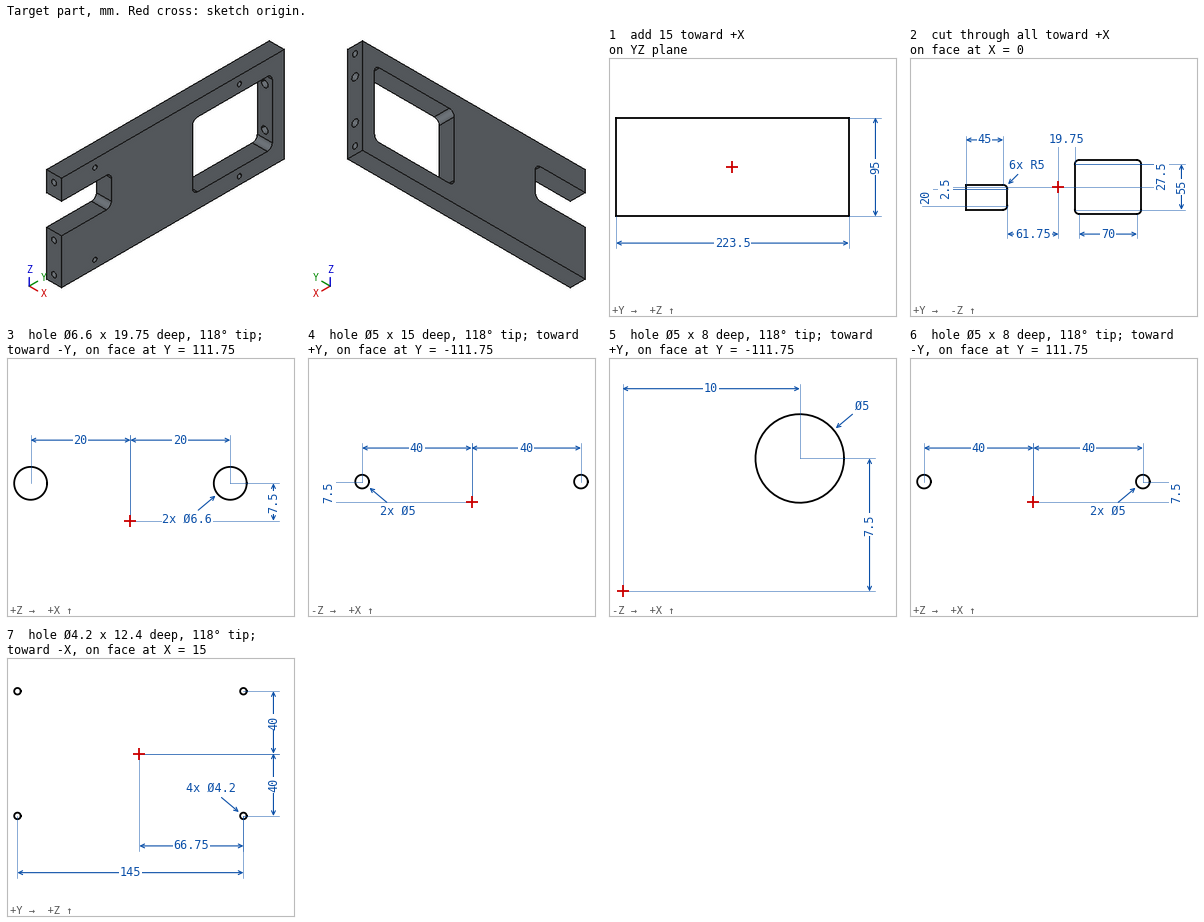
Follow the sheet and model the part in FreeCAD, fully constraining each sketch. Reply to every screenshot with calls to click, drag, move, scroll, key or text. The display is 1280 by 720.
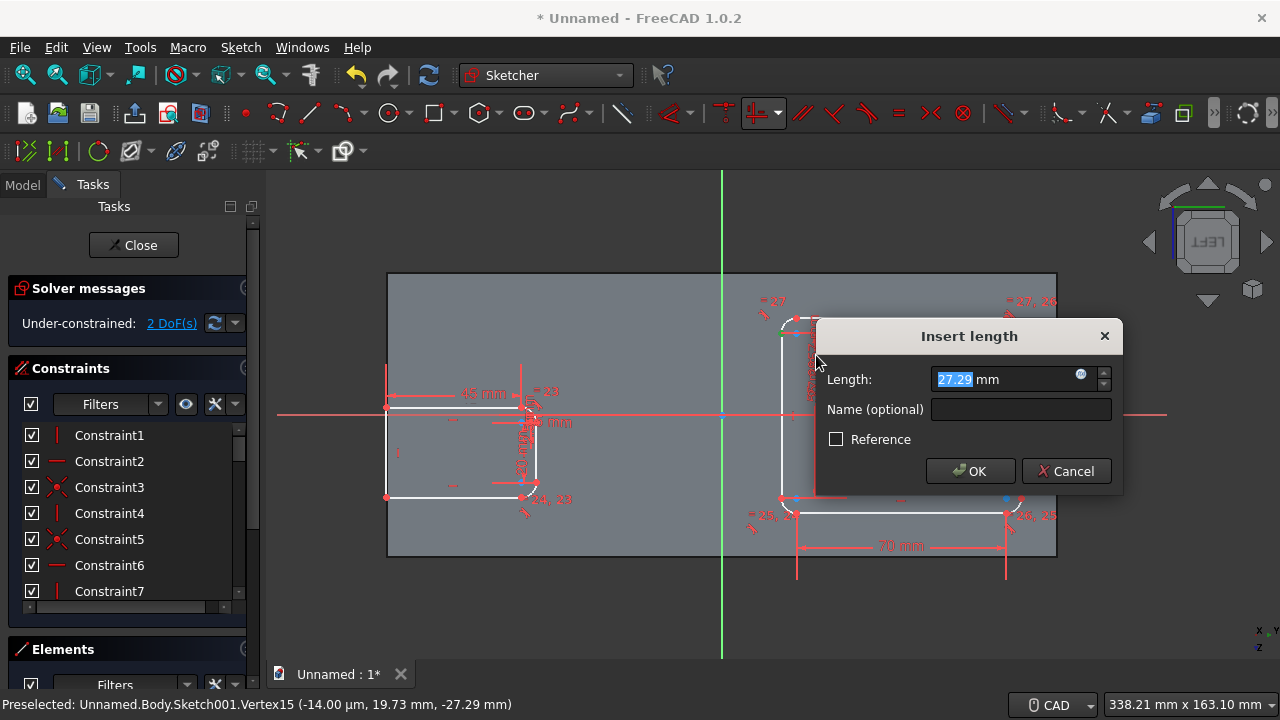
text(27.5)
key(Return)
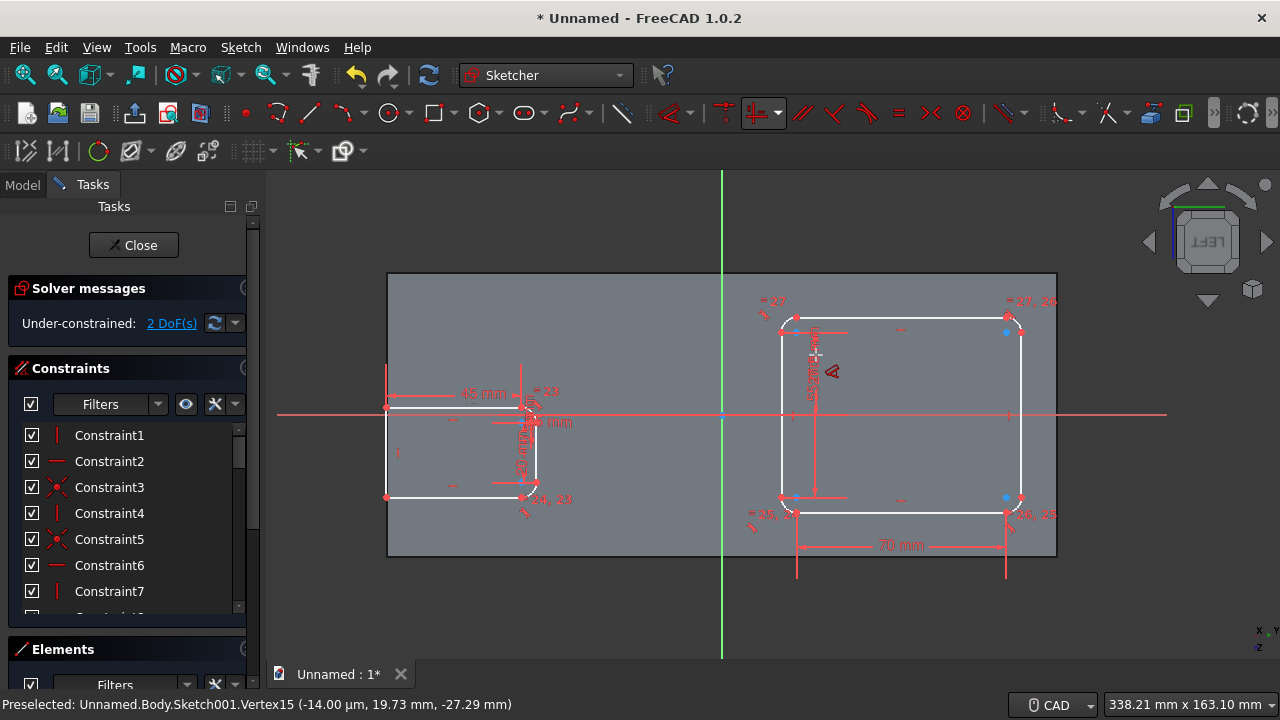
click(536, 483)
click(629, 517)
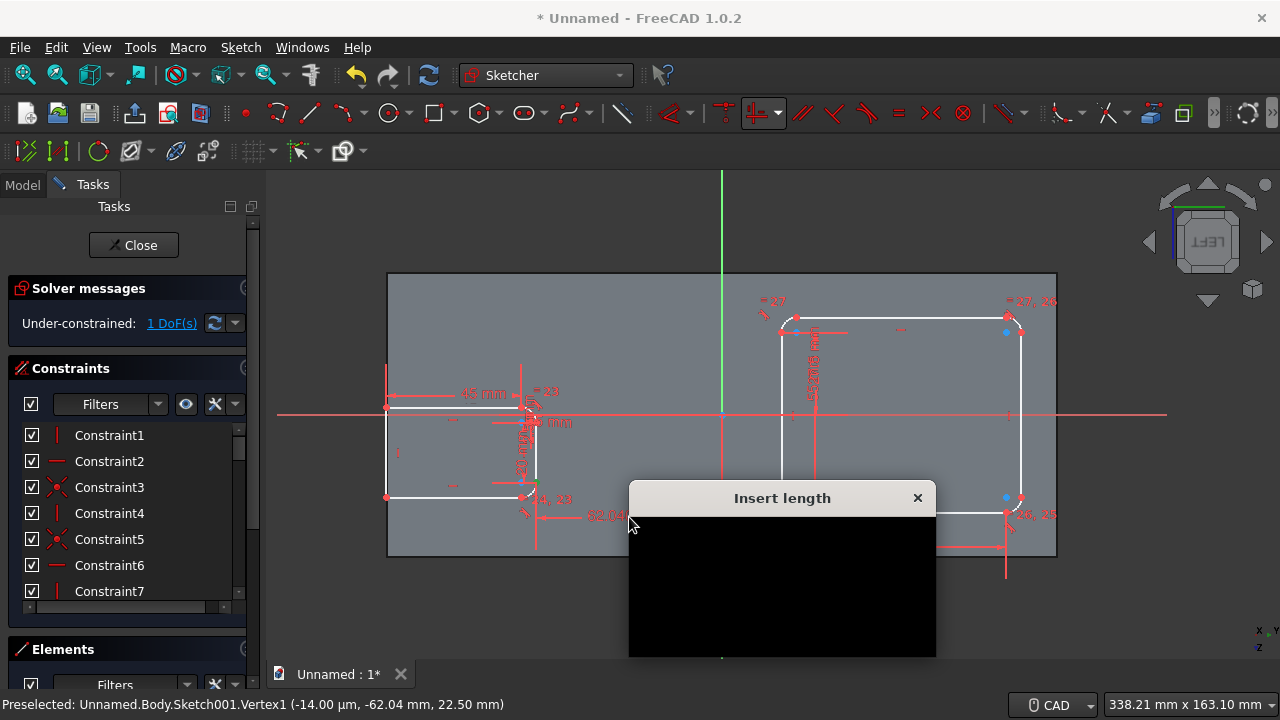
text(61.75)
key(Return)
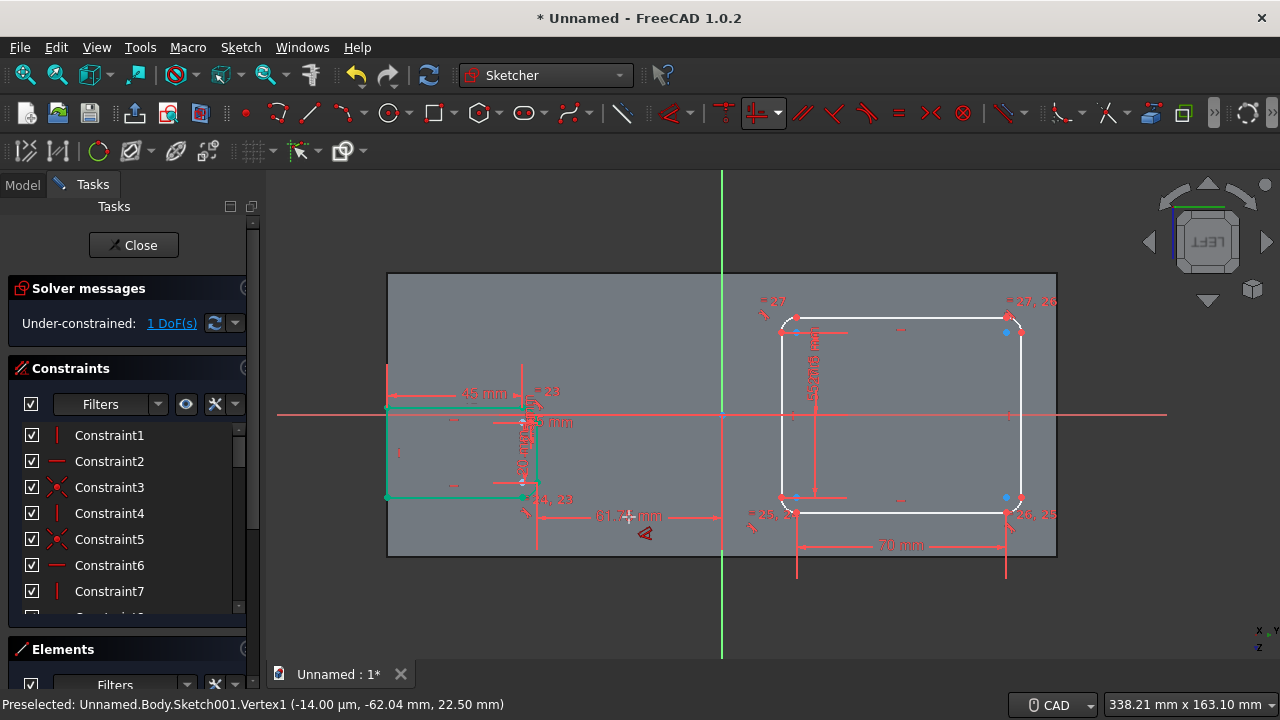
click(782, 333)
click(752, 299)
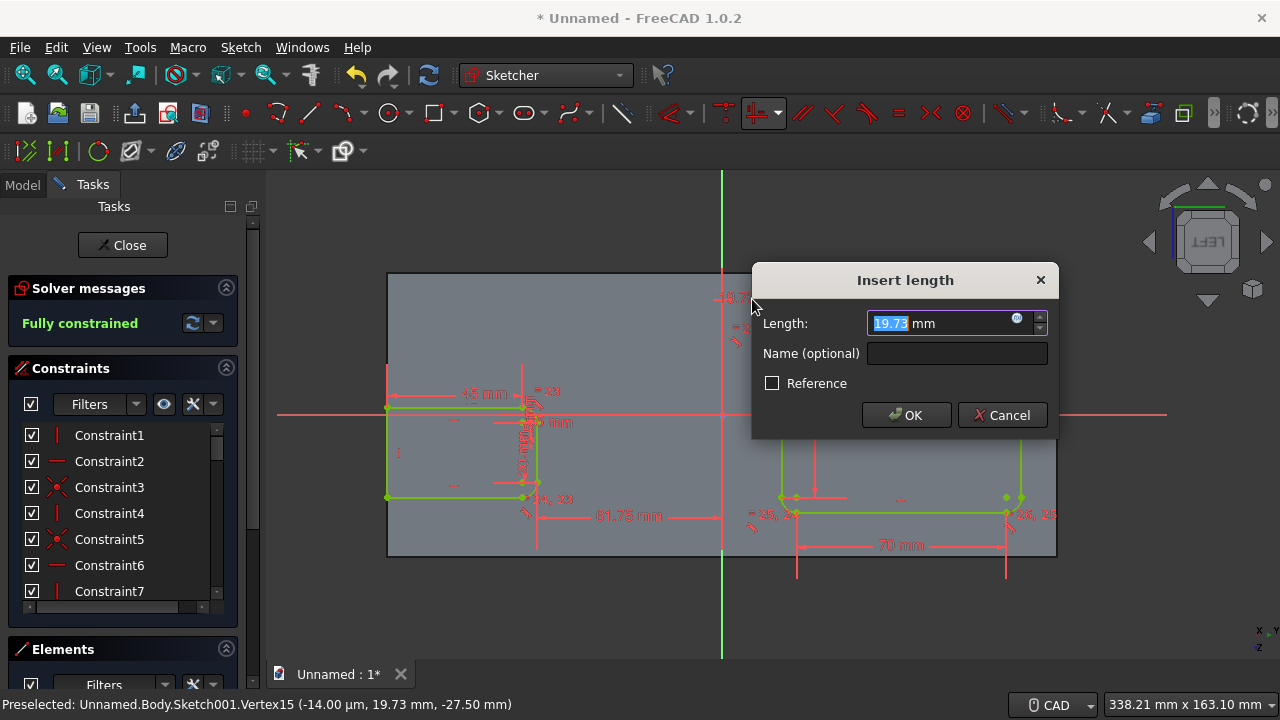
text(19.75)
key(Return)
key(Escape)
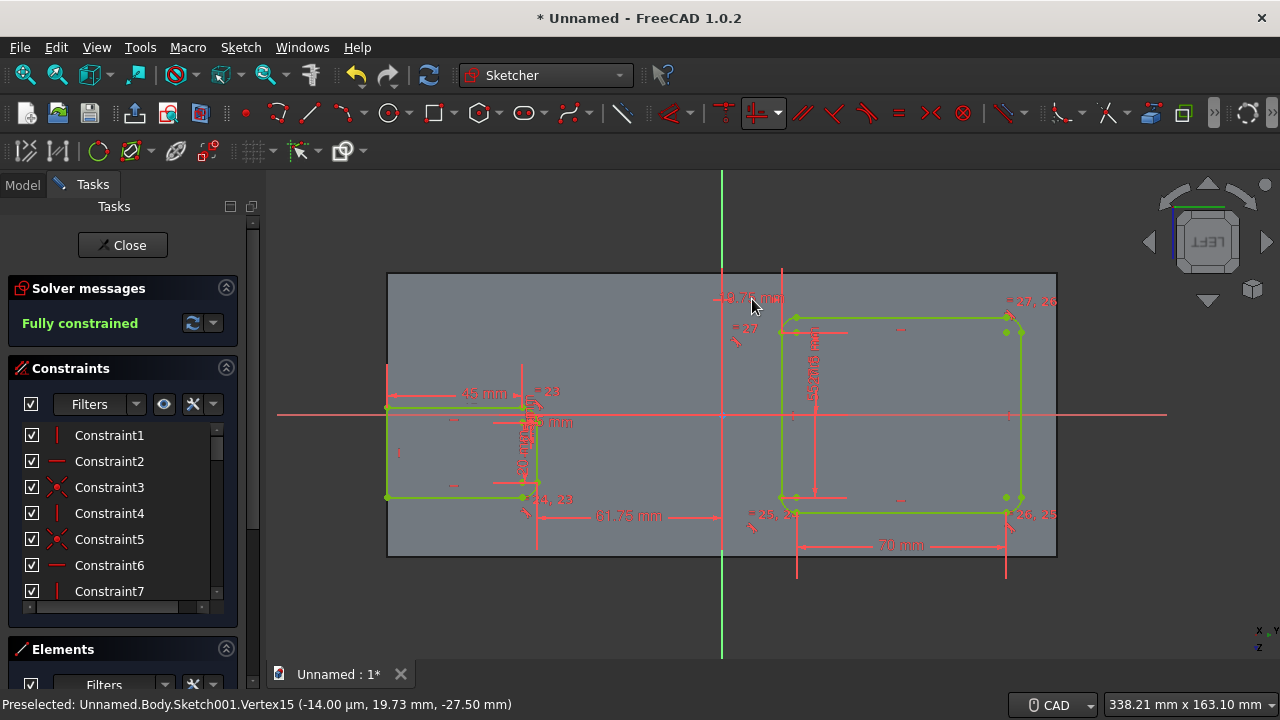
click(123, 245)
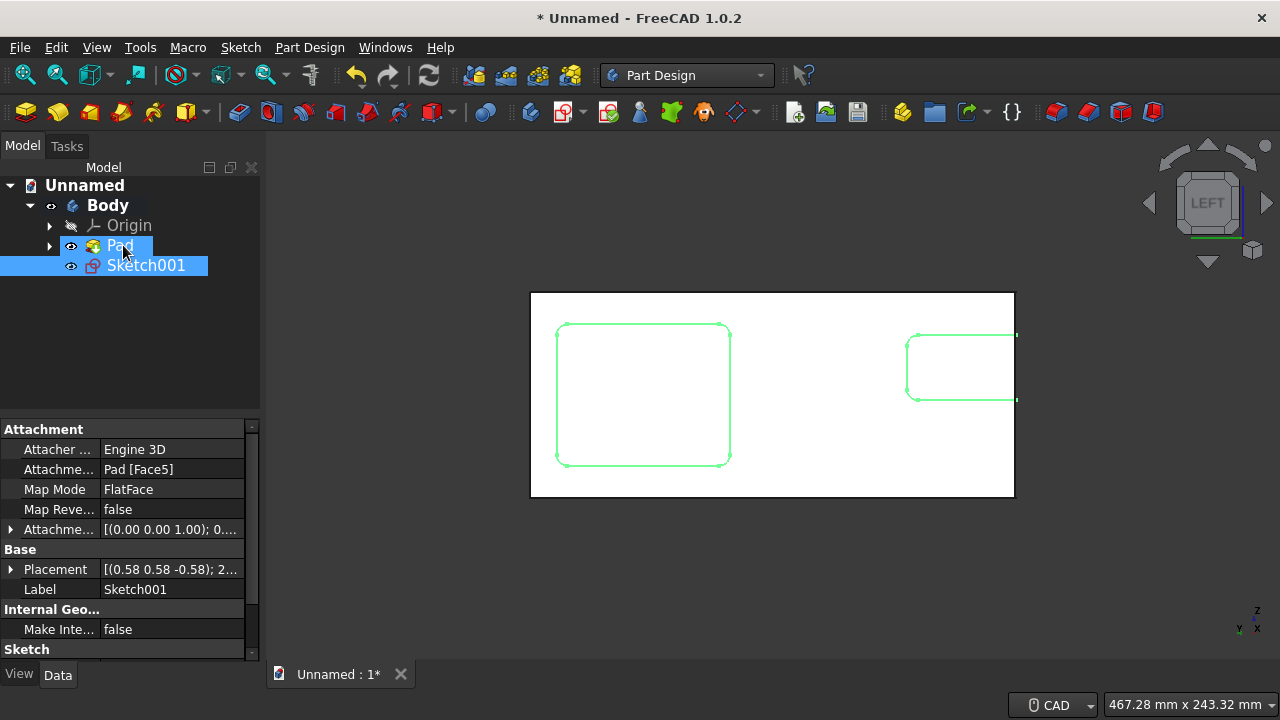
click(240, 112)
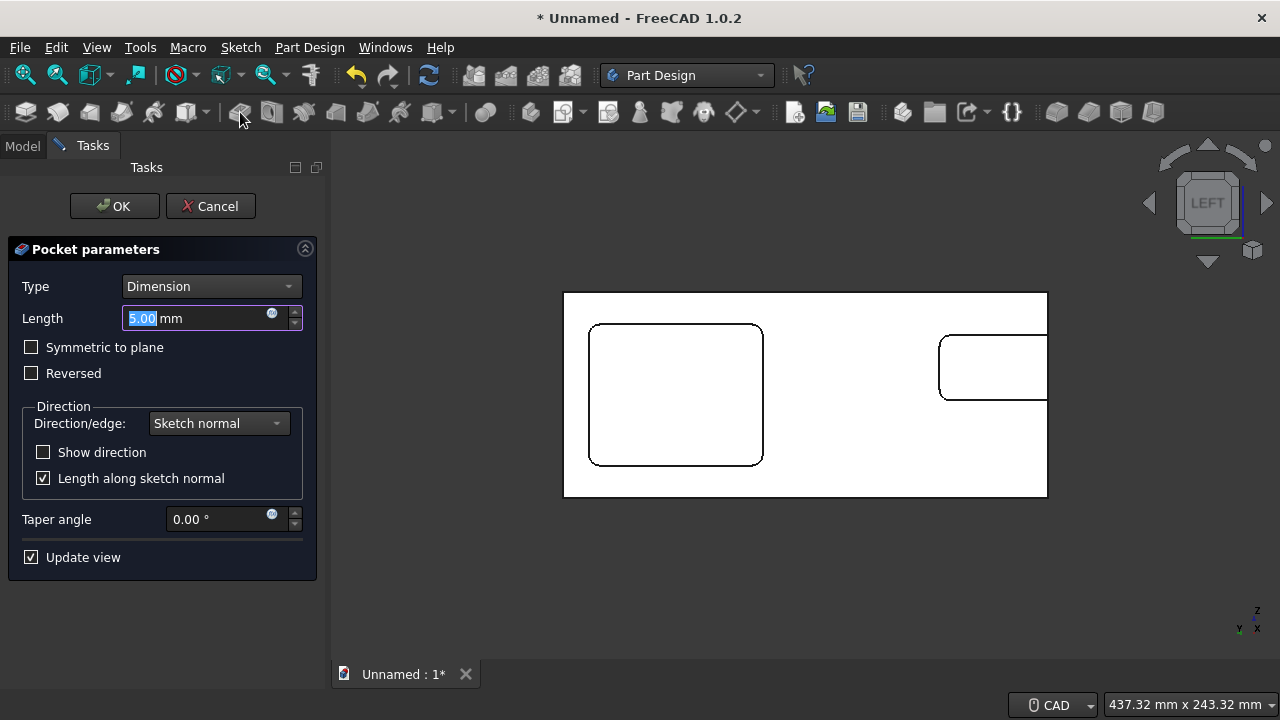
click(212, 286)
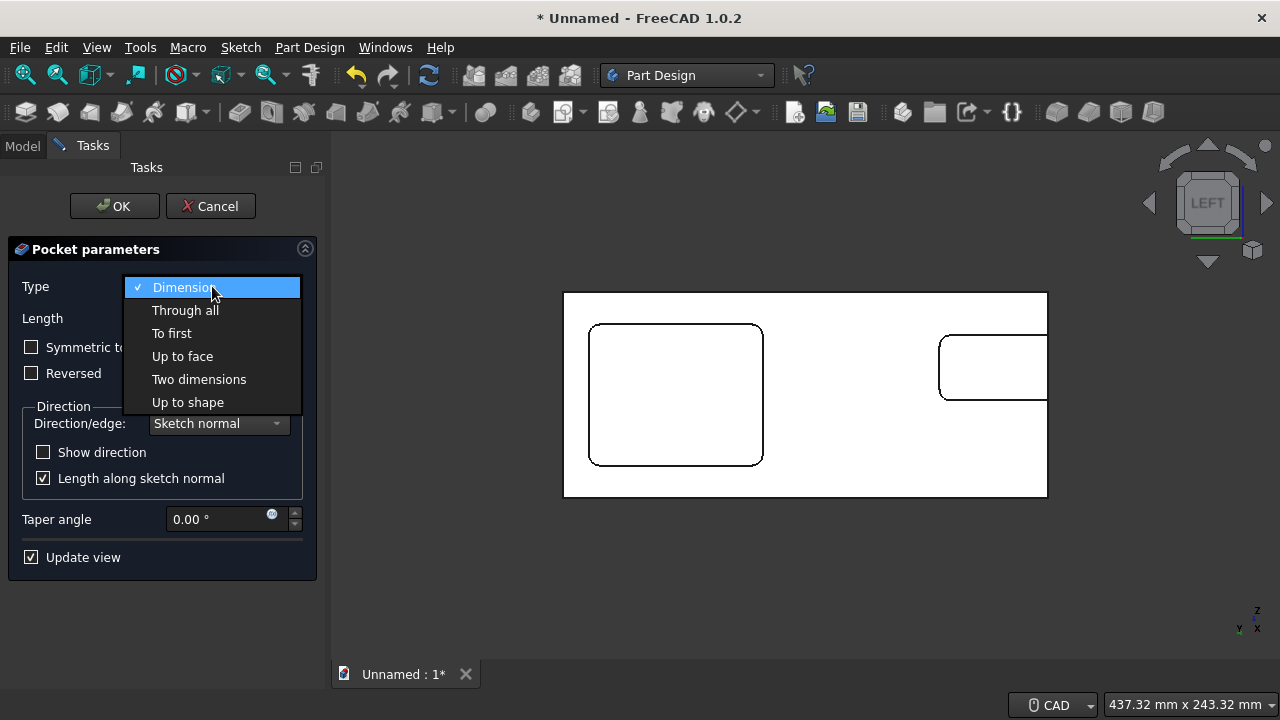
click(212, 310)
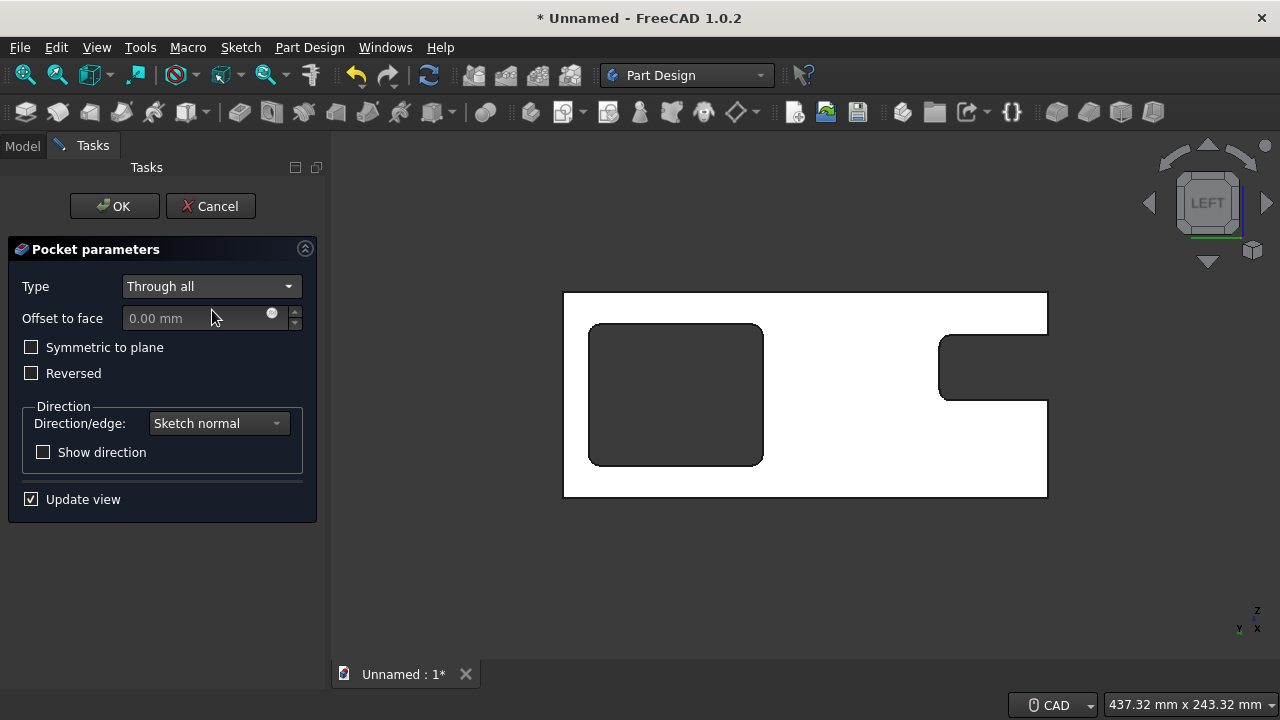
click(115, 206)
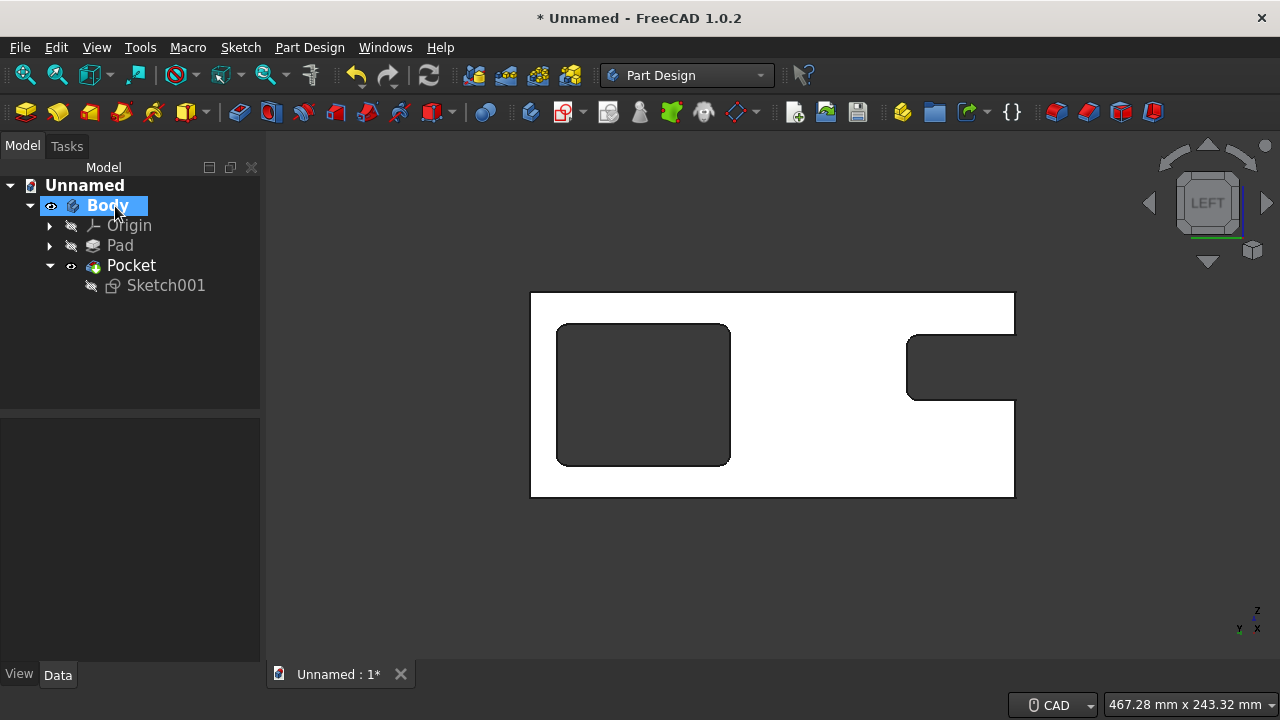
key(4)